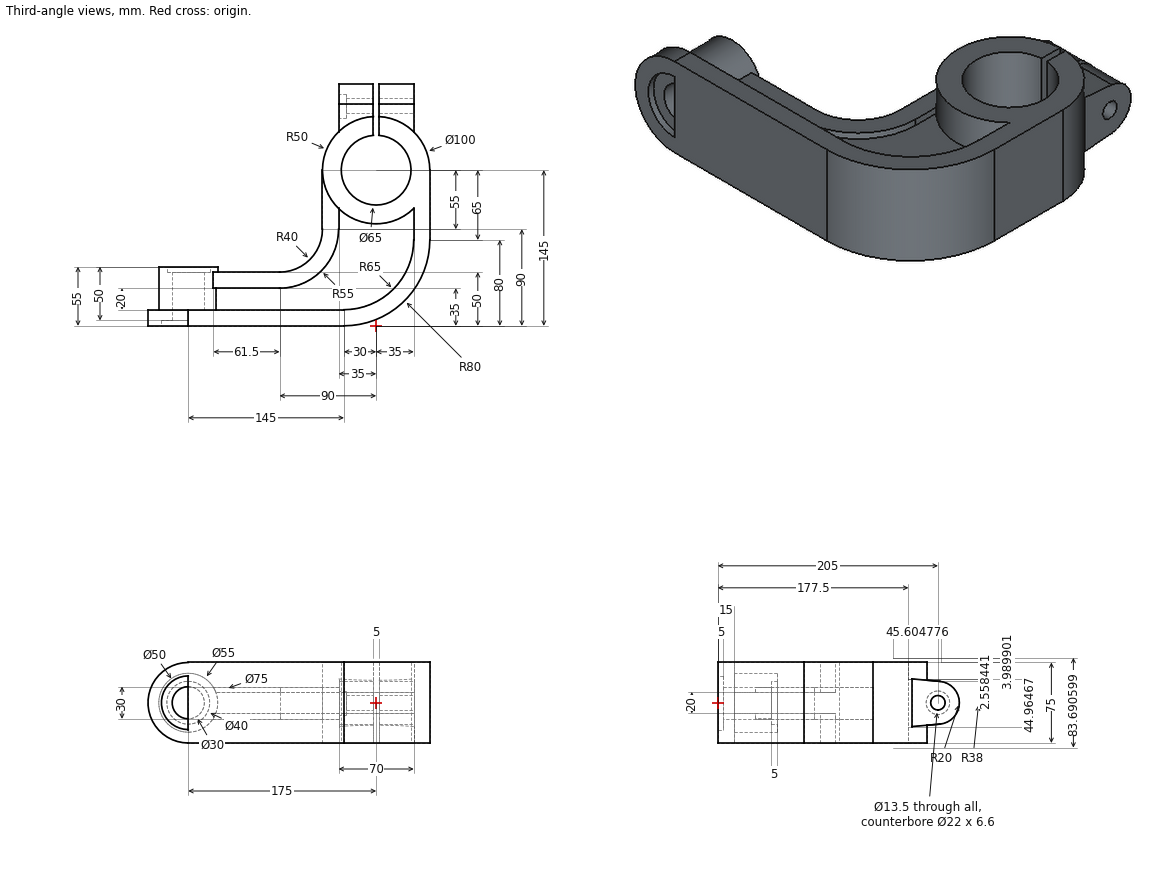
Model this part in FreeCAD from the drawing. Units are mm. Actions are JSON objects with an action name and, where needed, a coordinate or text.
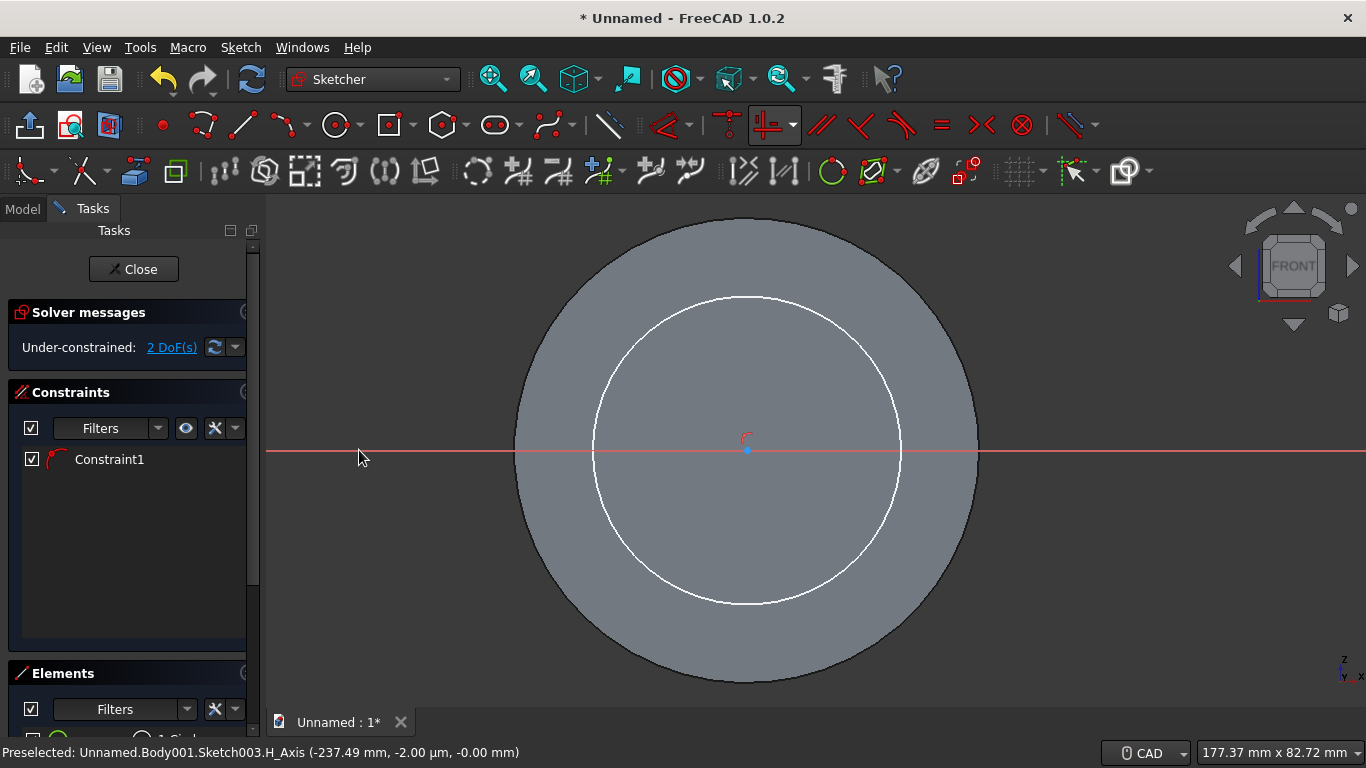
{"action": "key", "text": "d"}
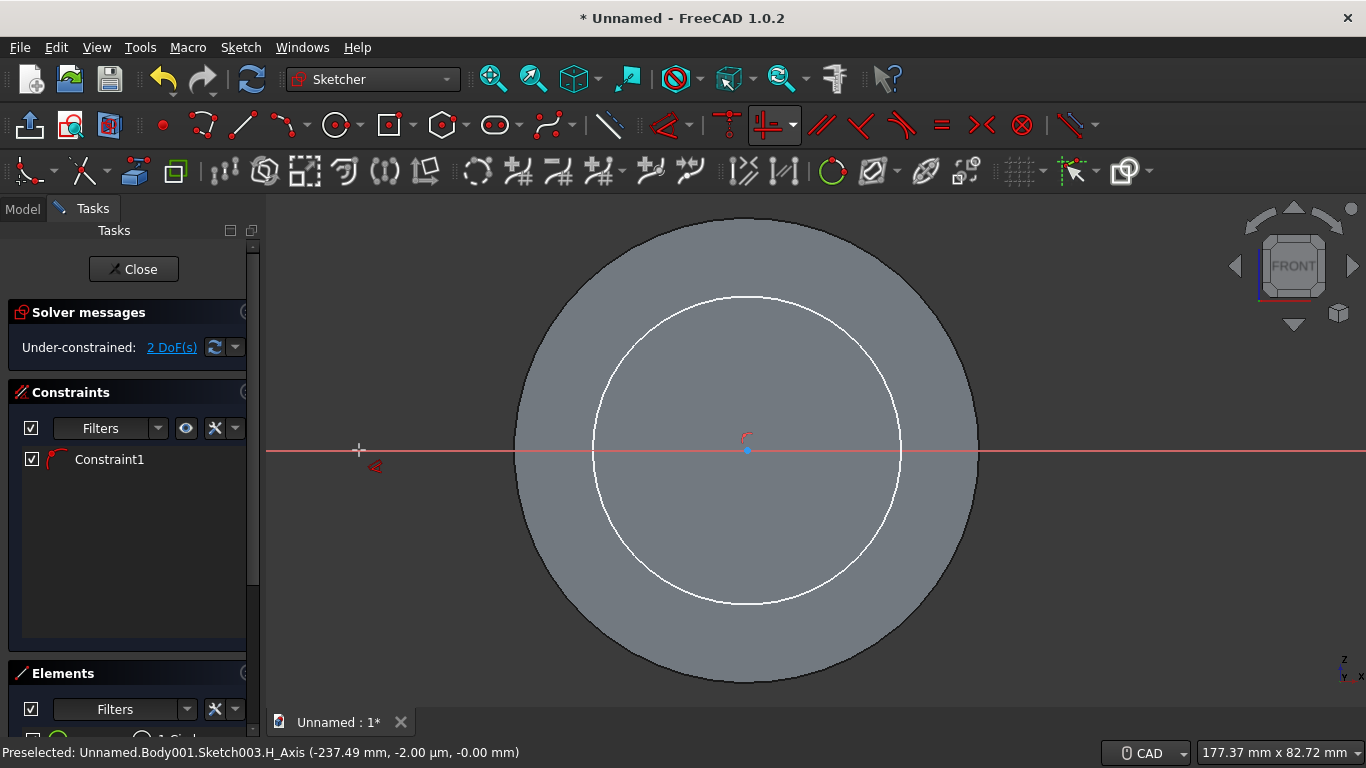
{"action": "left_click", "coordinate": [856, 341]}
{"action": "left_click", "coordinate": [879, 318]}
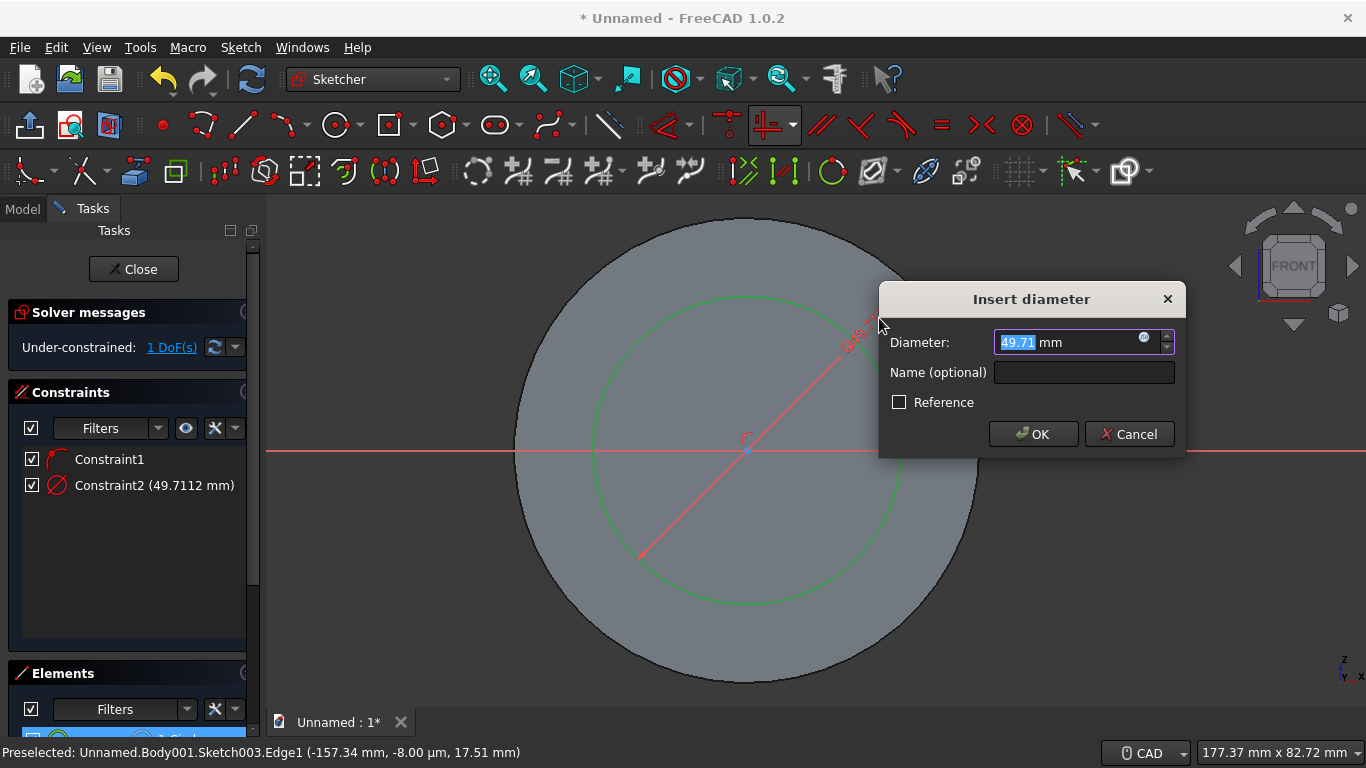
{"action": "type", "text": "50"}
{"action": "key", "text": "Return"}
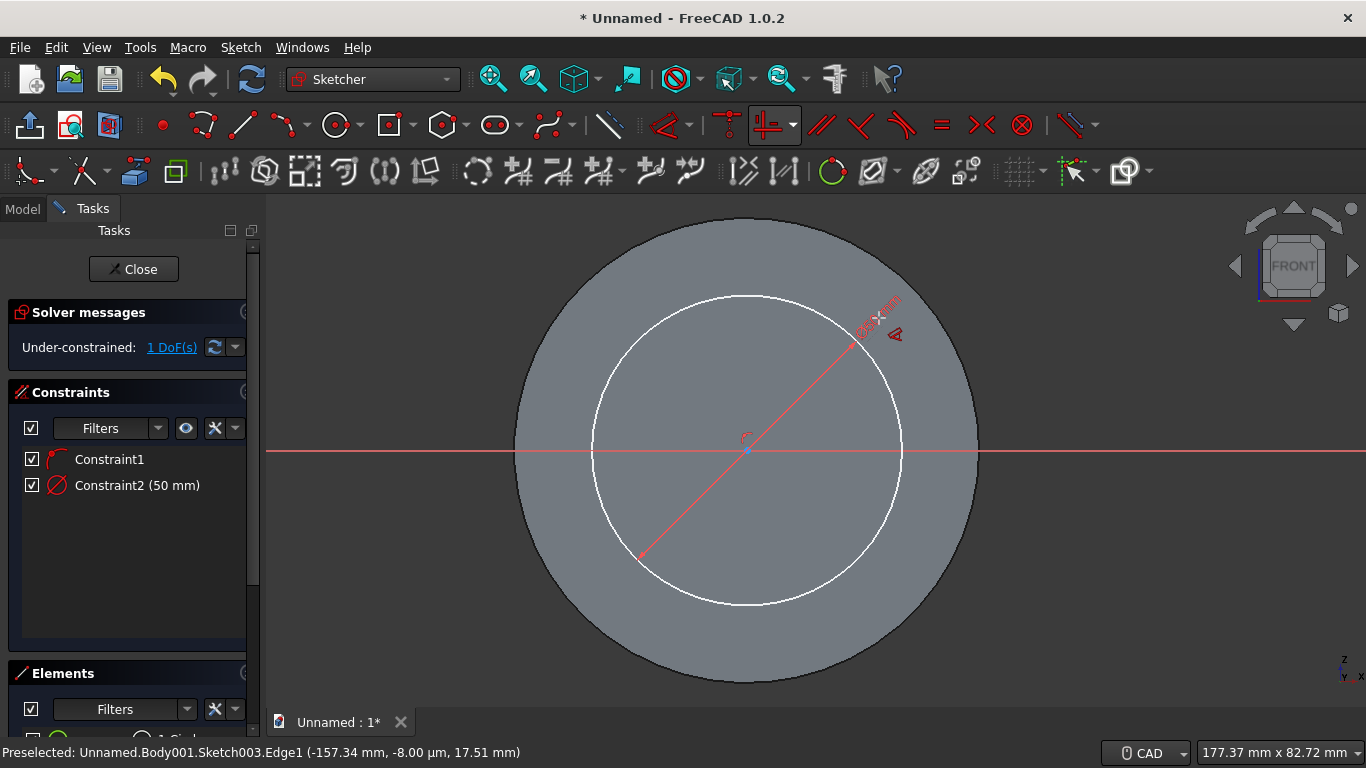
{"action": "left_click", "coordinate": [747, 450]}
{"action": "left_click", "coordinate": [974, 484]}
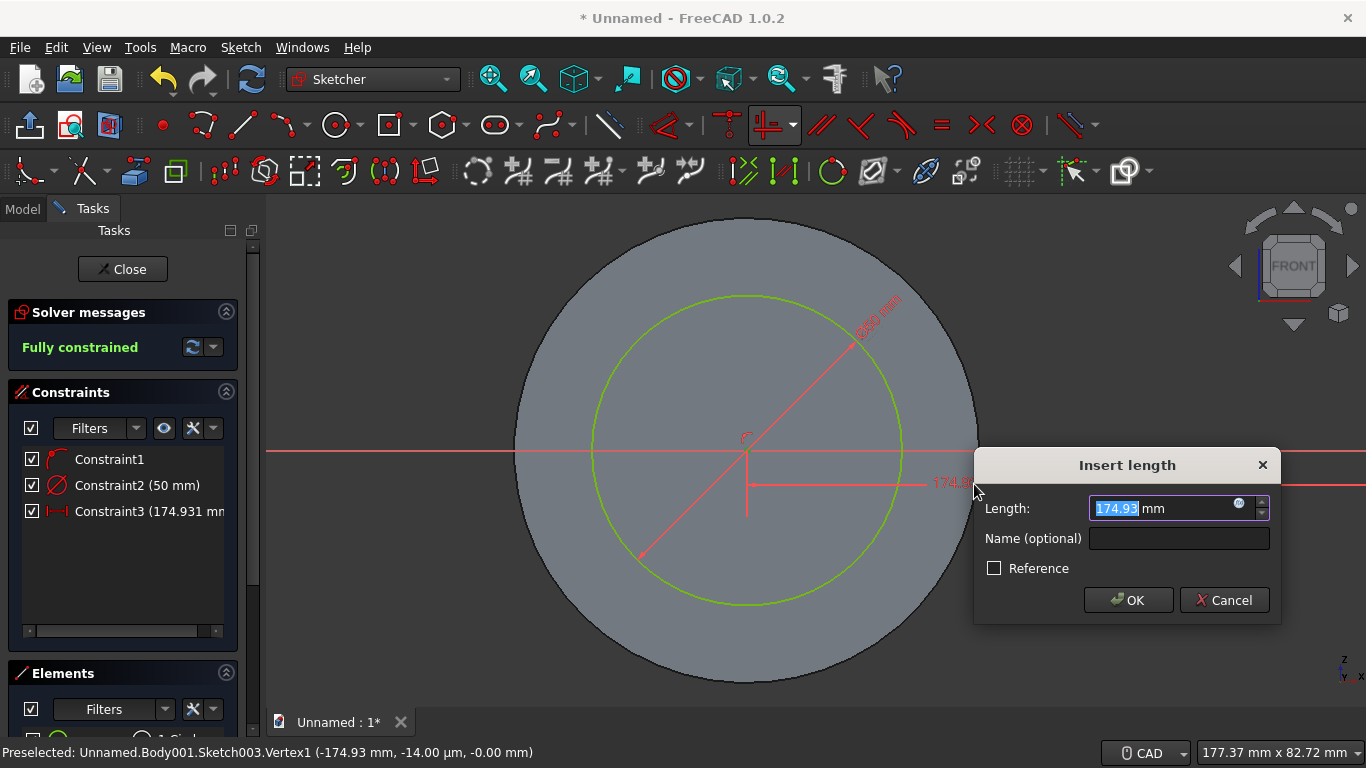
{"action": "type", "text": "175"}
{"action": "key", "text": "Return"}
{"action": "key", "text": "Escape"}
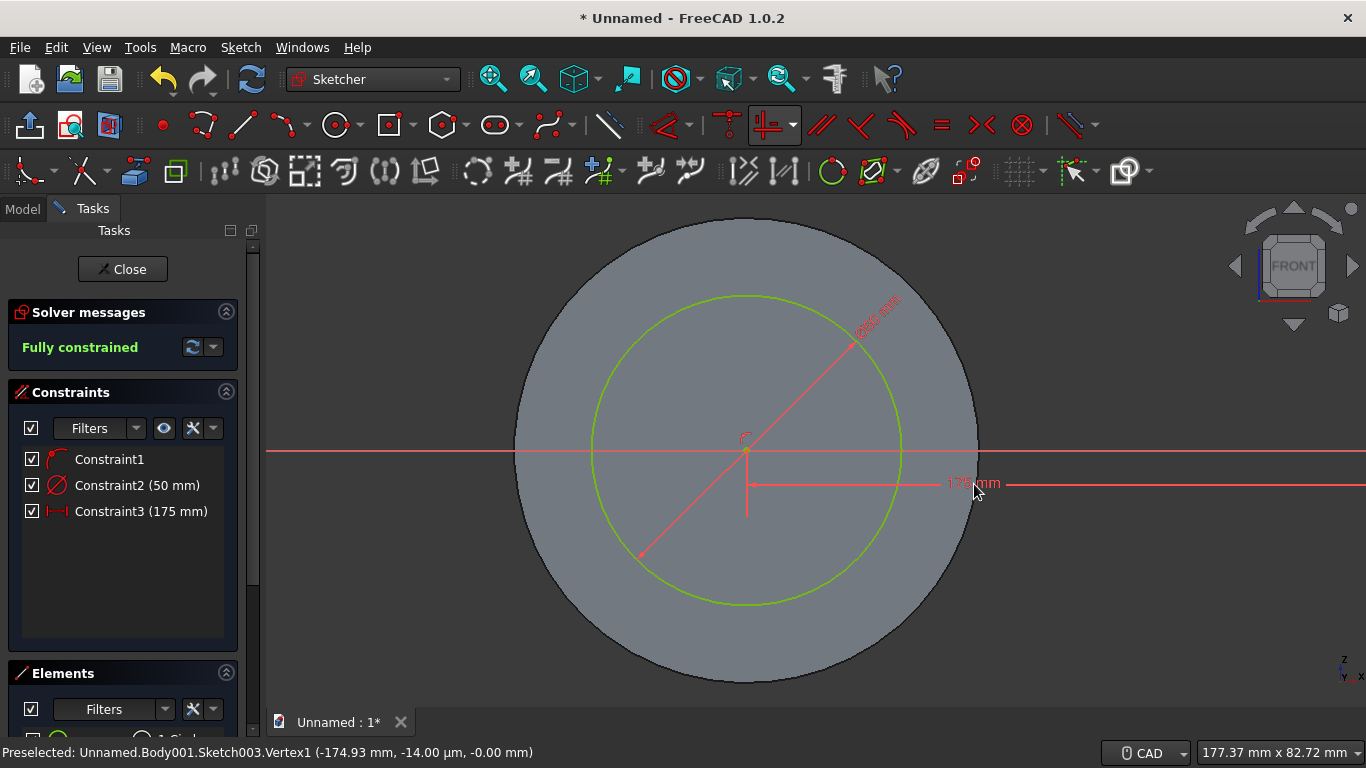
{"action": "left_click", "coordinate": [123, 269]}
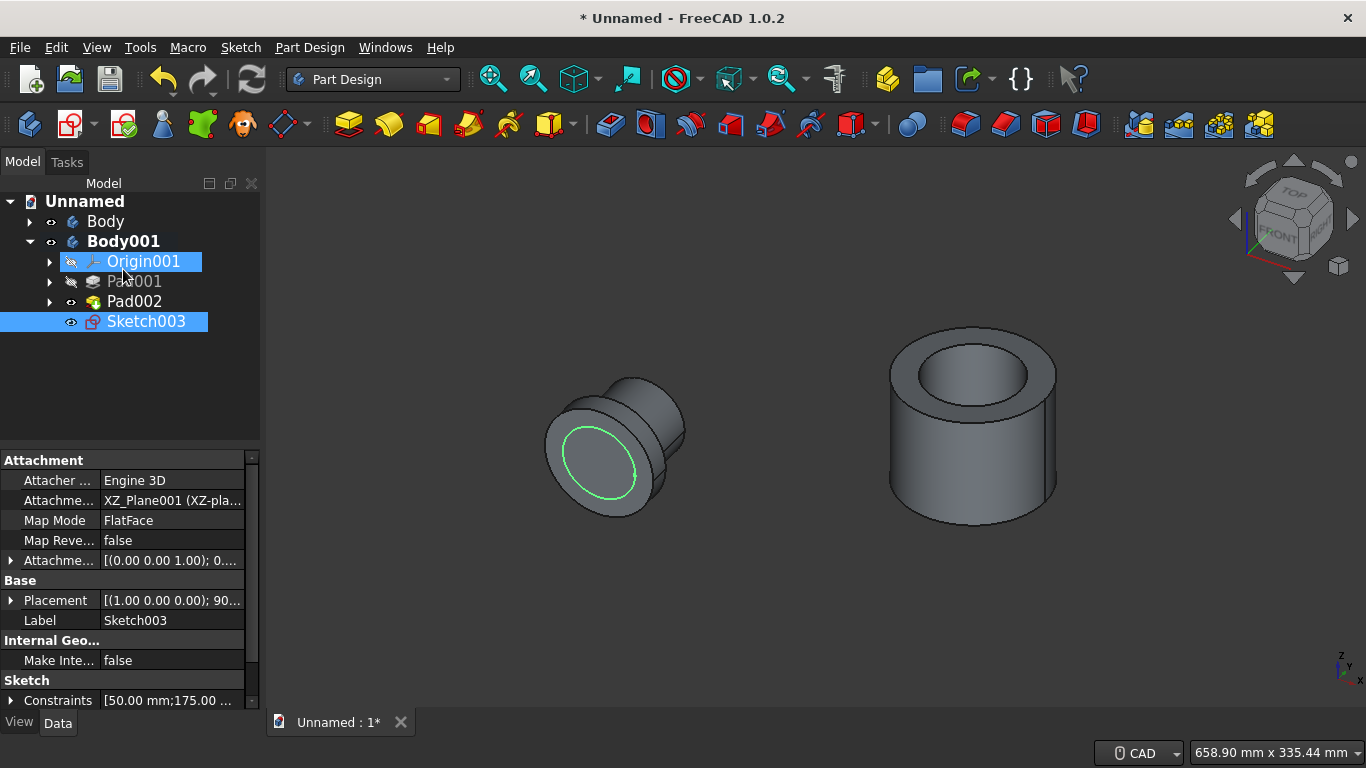
{"action": "left_click", "coordinate": [612, 124]}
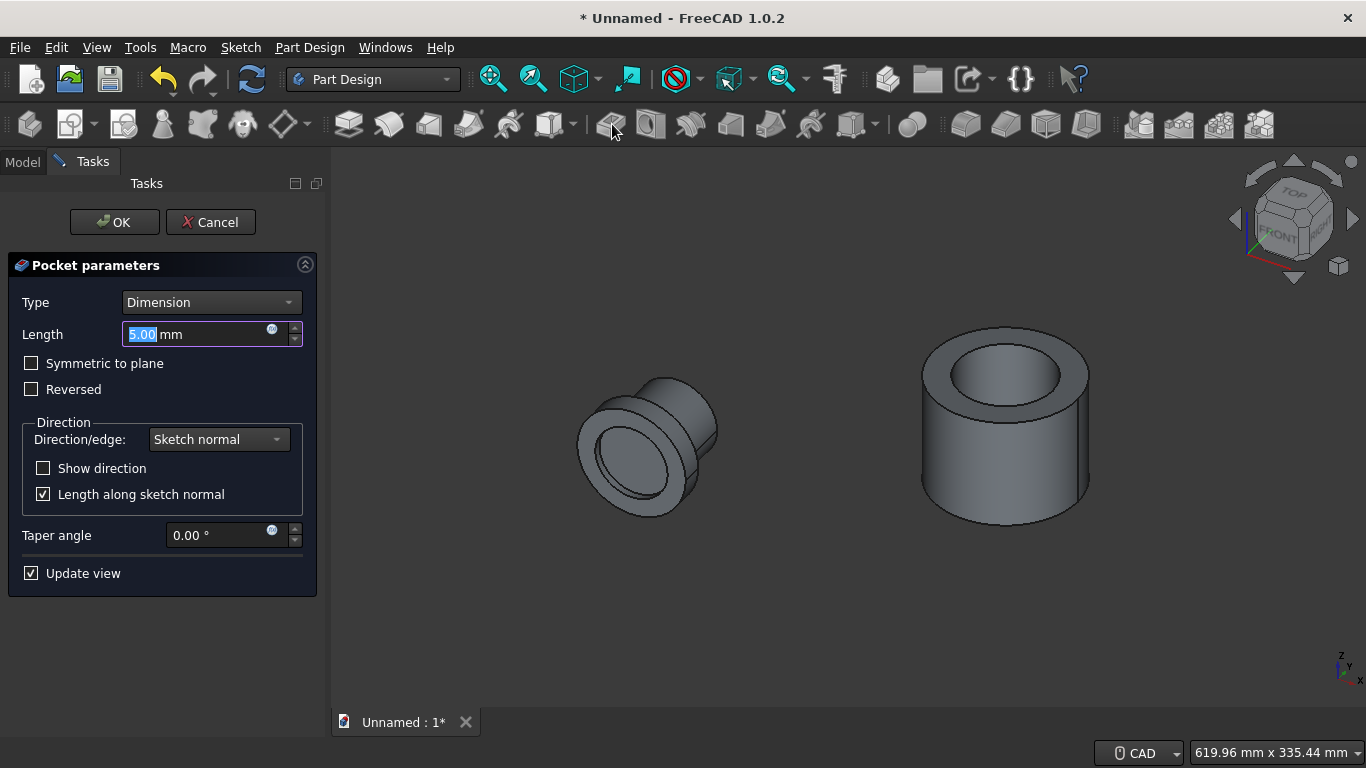
{"action": "type", "text": "5"}
{"action": "key", "text": "Tab"}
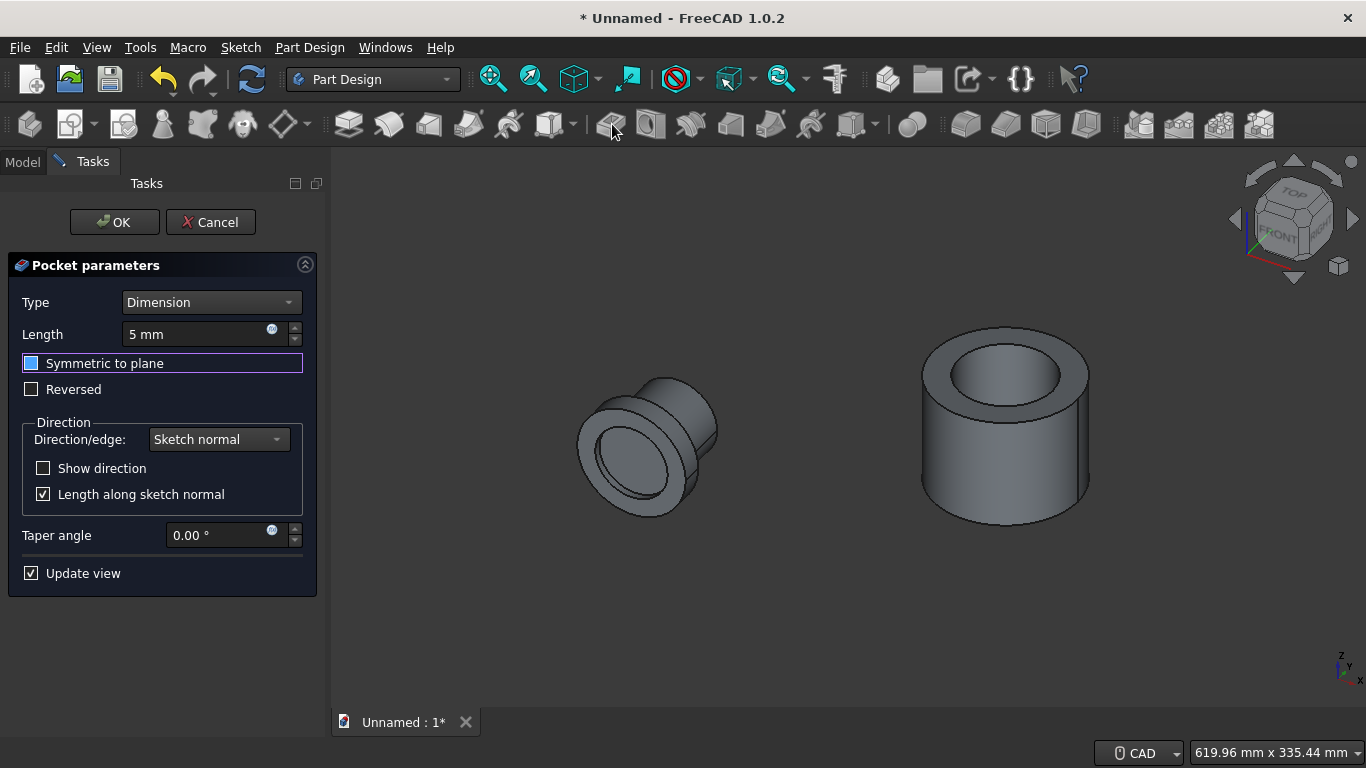
{"action": "left_click", "coordinate": [115, 222]}